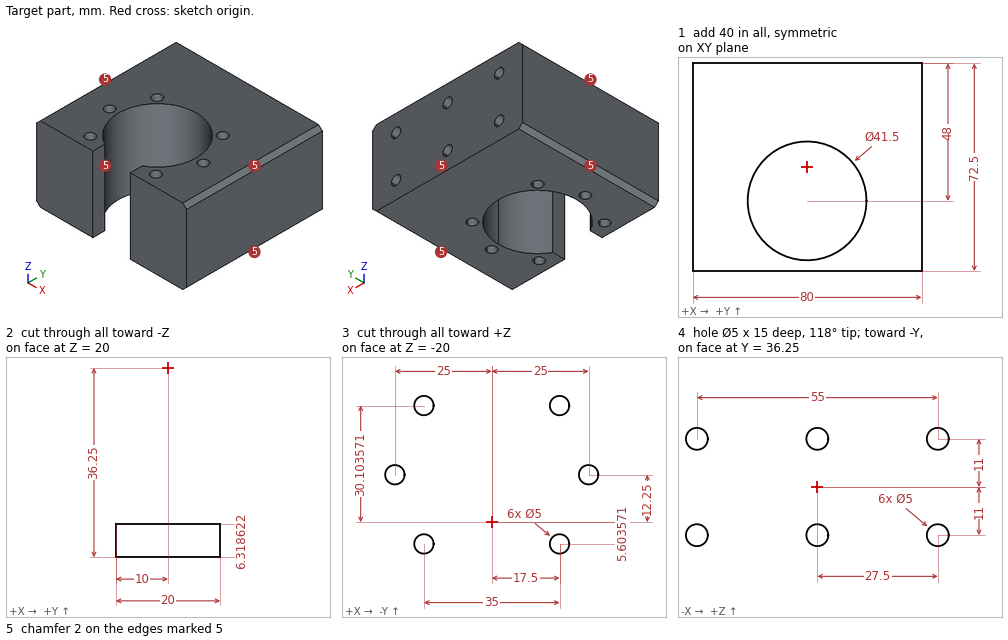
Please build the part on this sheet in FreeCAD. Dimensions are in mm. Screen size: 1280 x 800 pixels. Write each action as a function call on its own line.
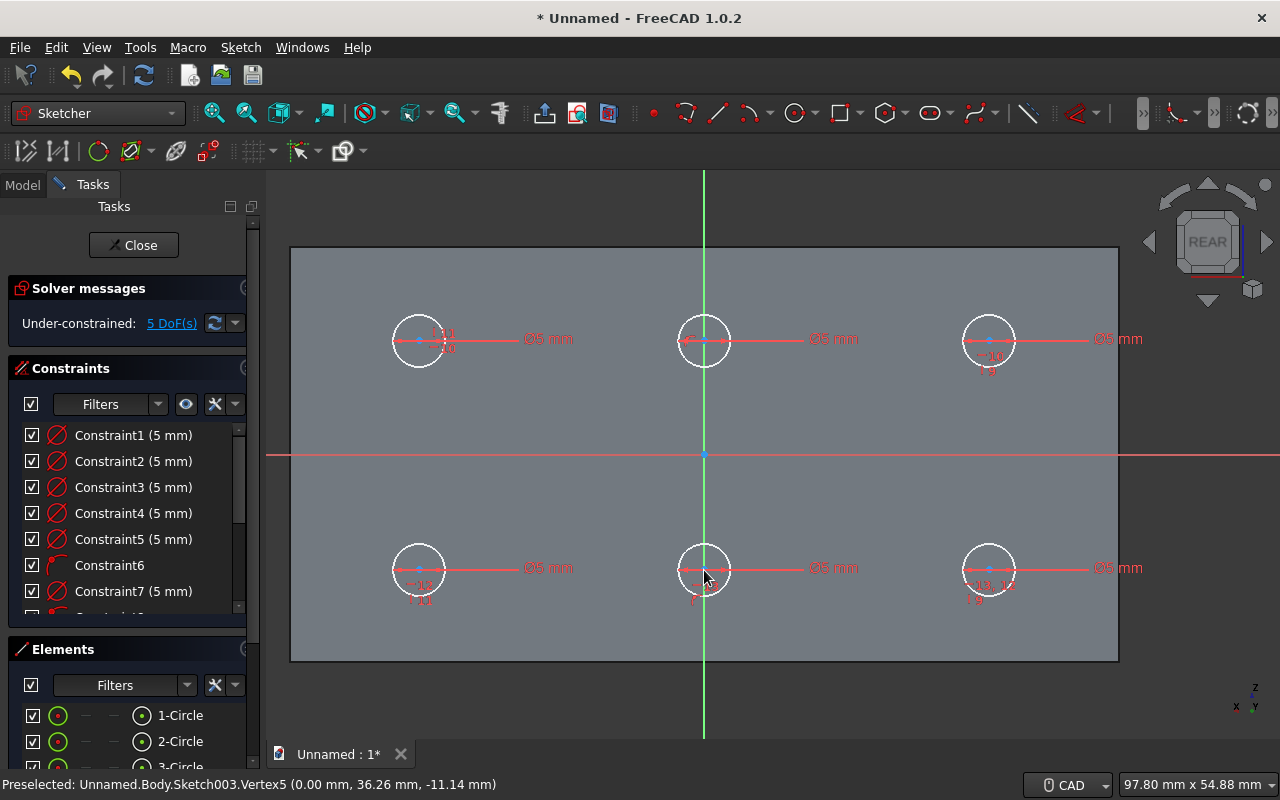
click(989, 341)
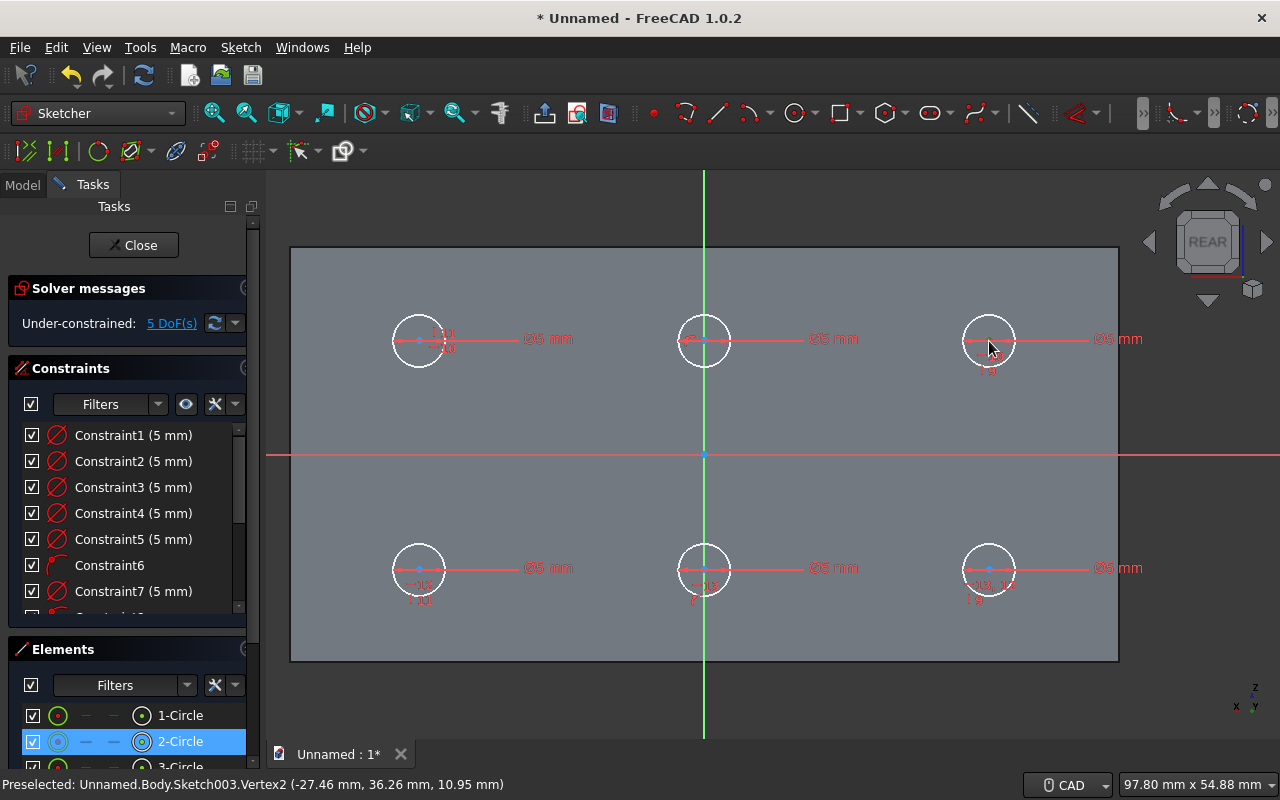
click(704, 341)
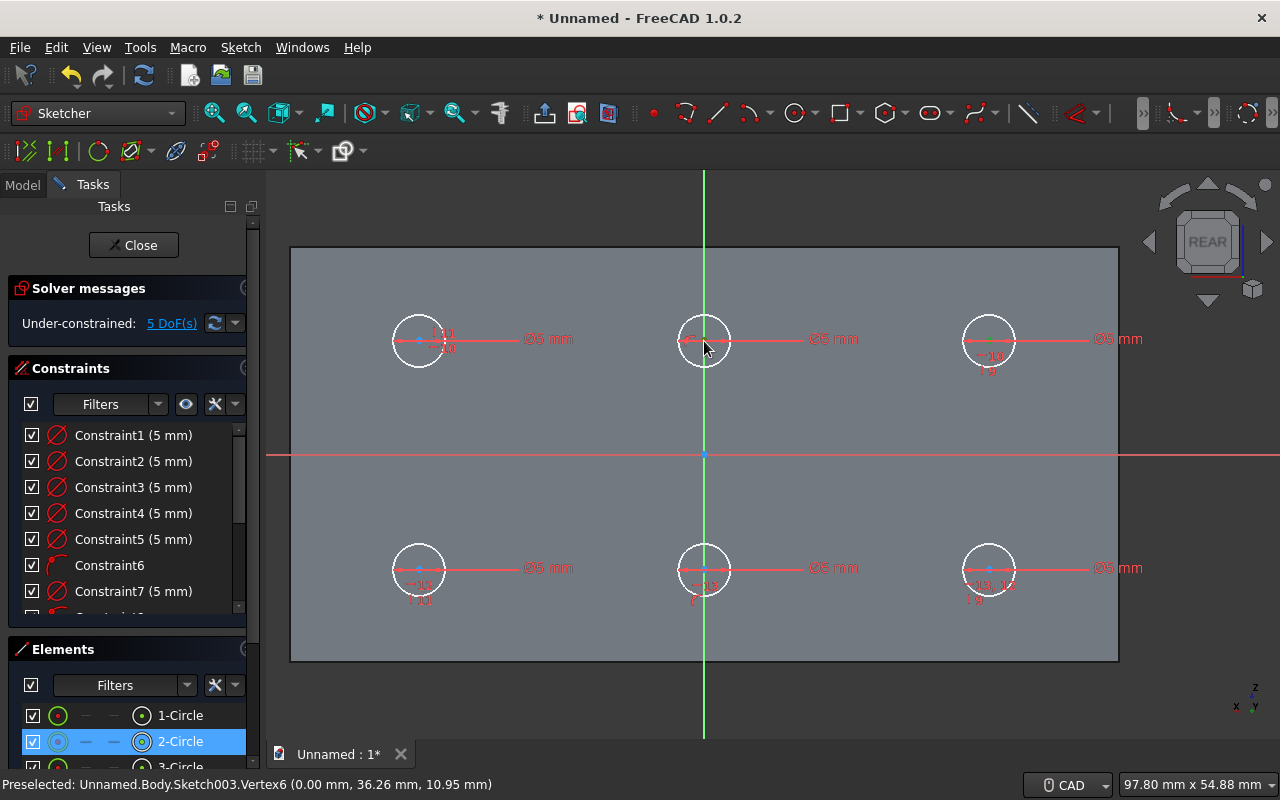
key(h)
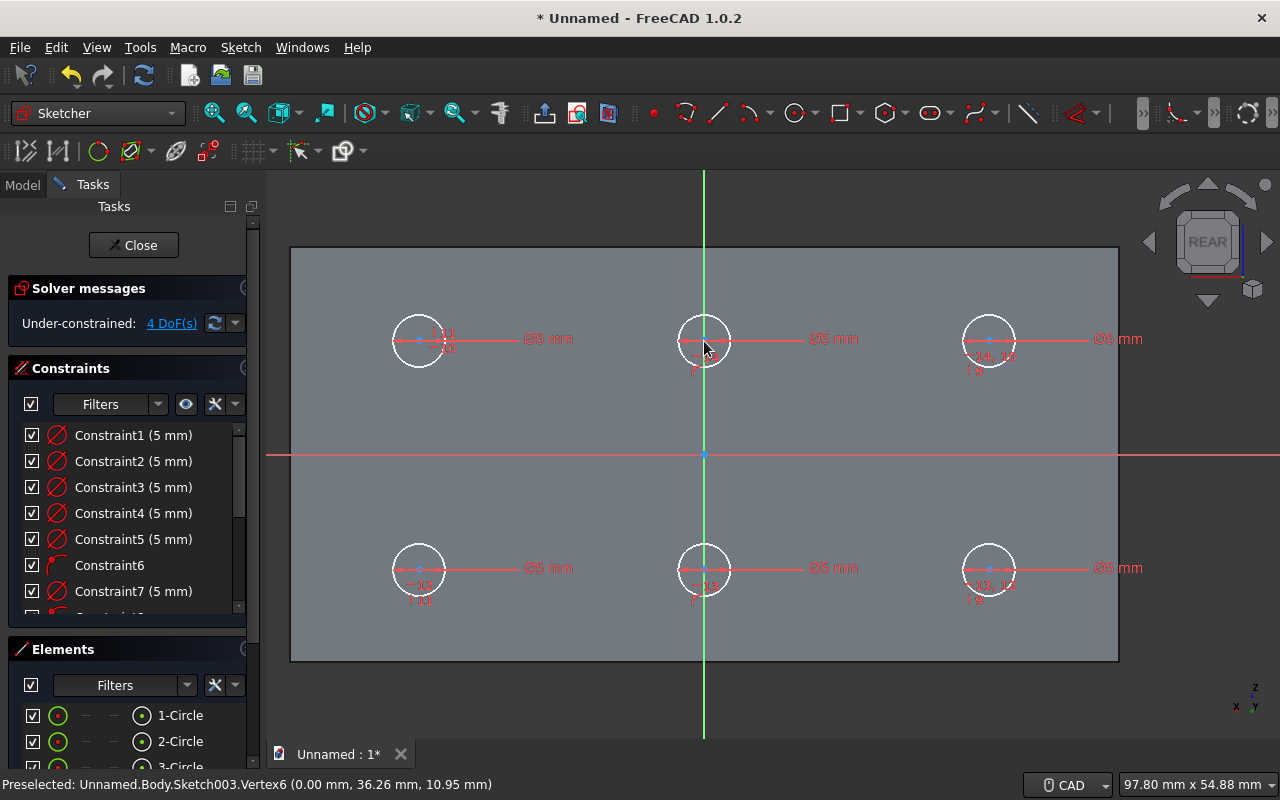
click(1076, 114)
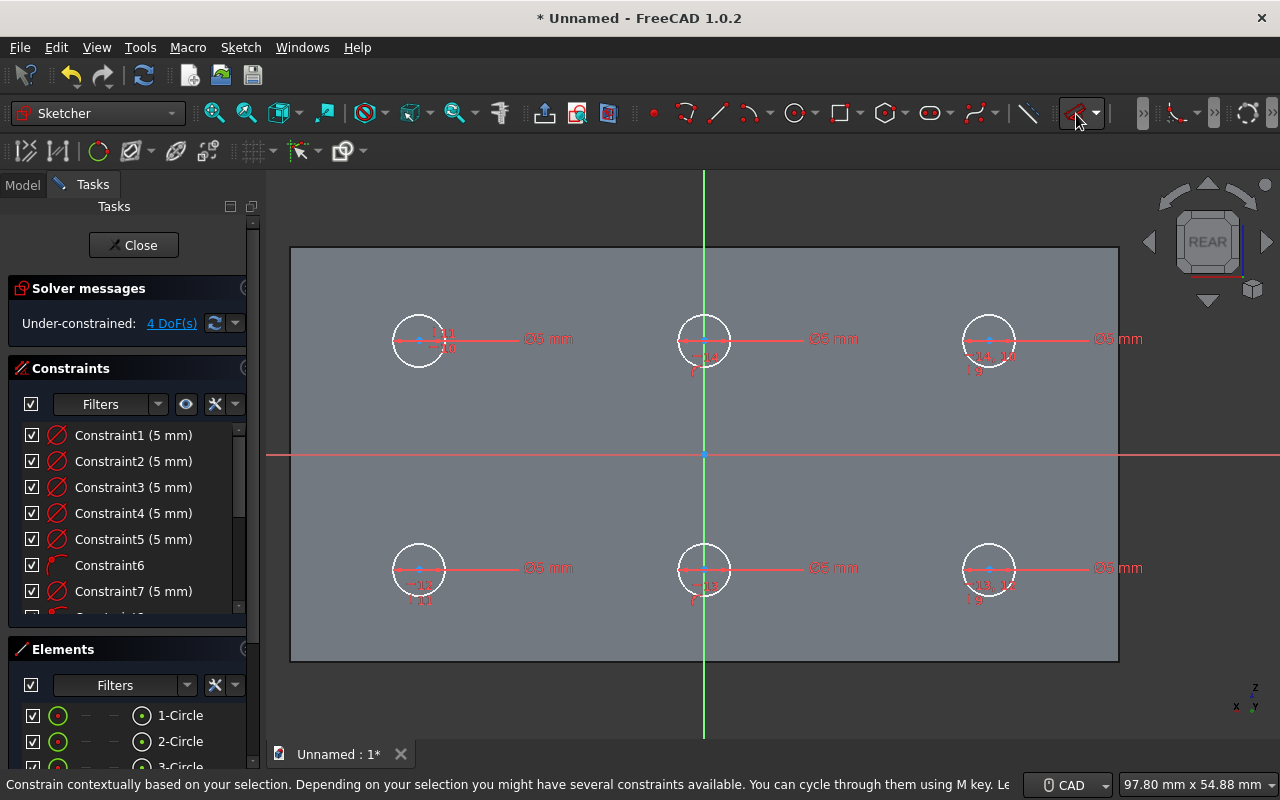
click(989, 570)
click(1023, 512)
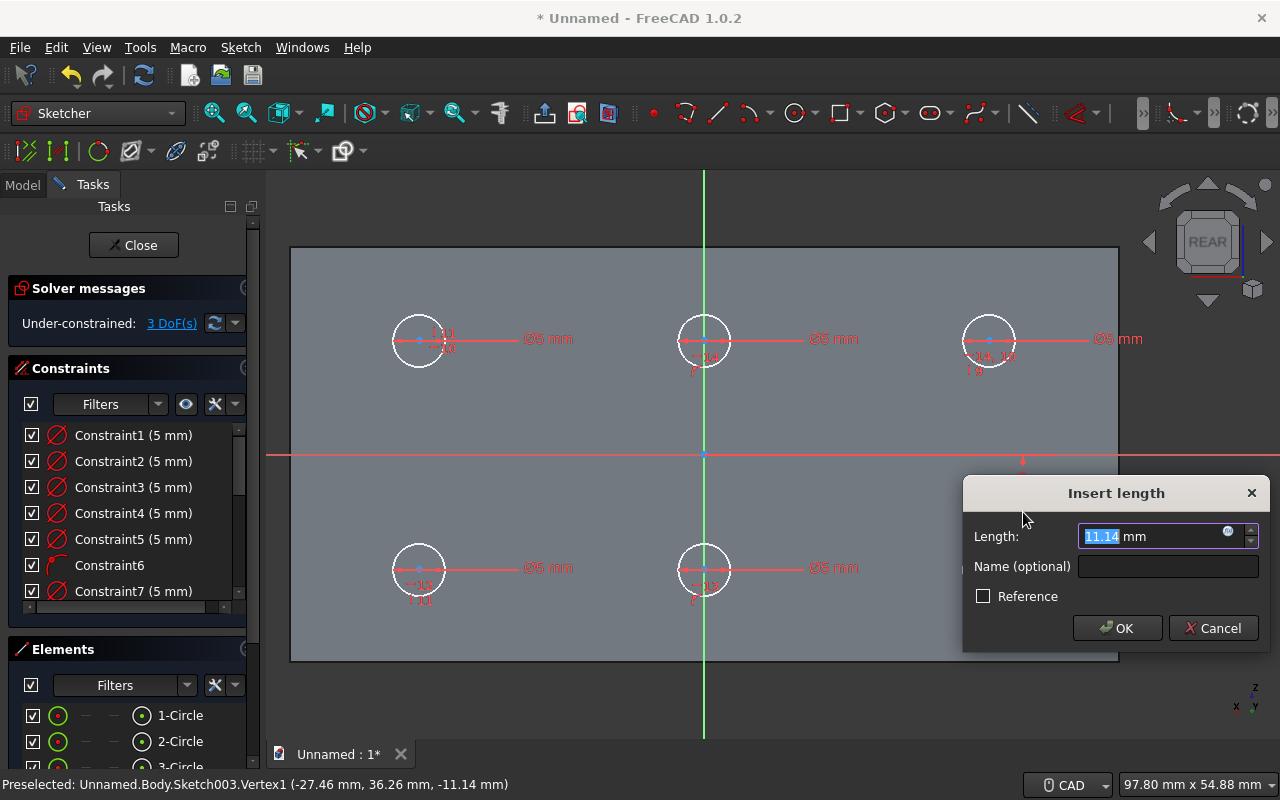
text(11)
key(Return)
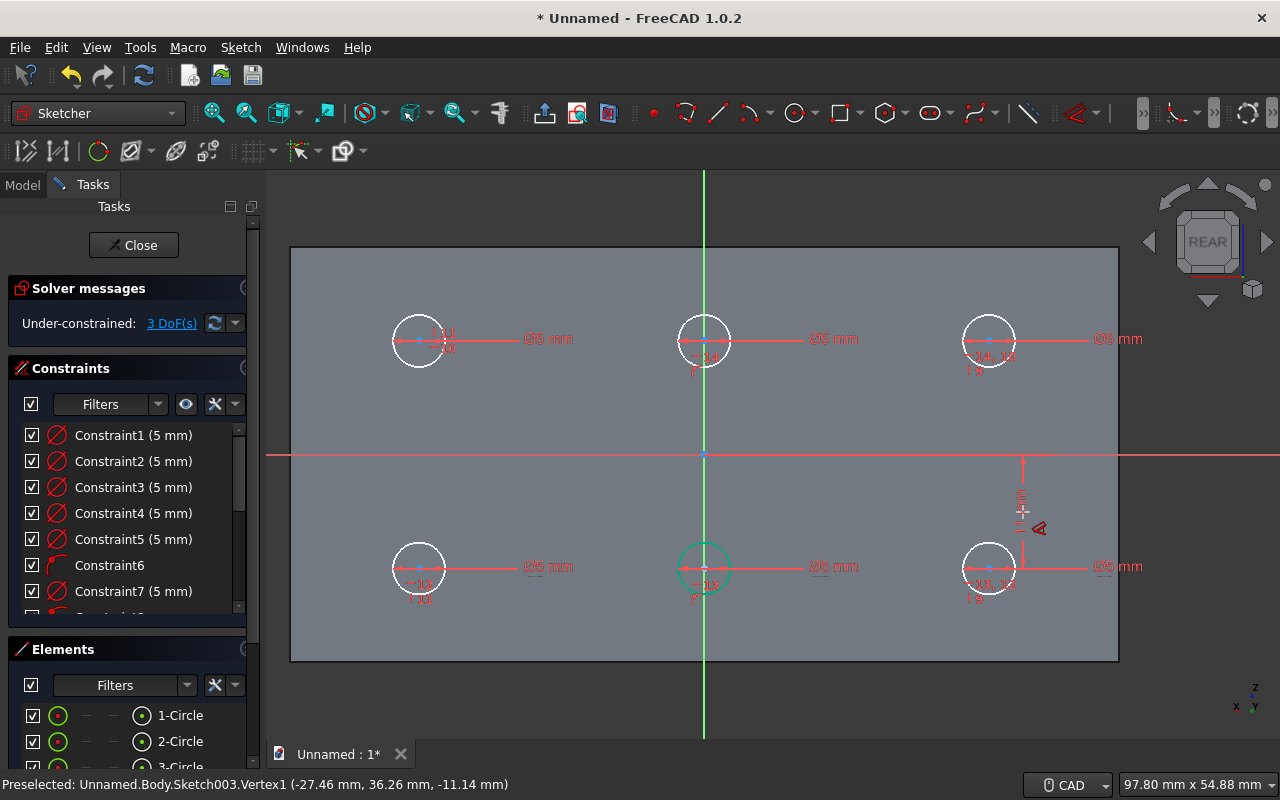
click(989, 341)
click(1023, 398)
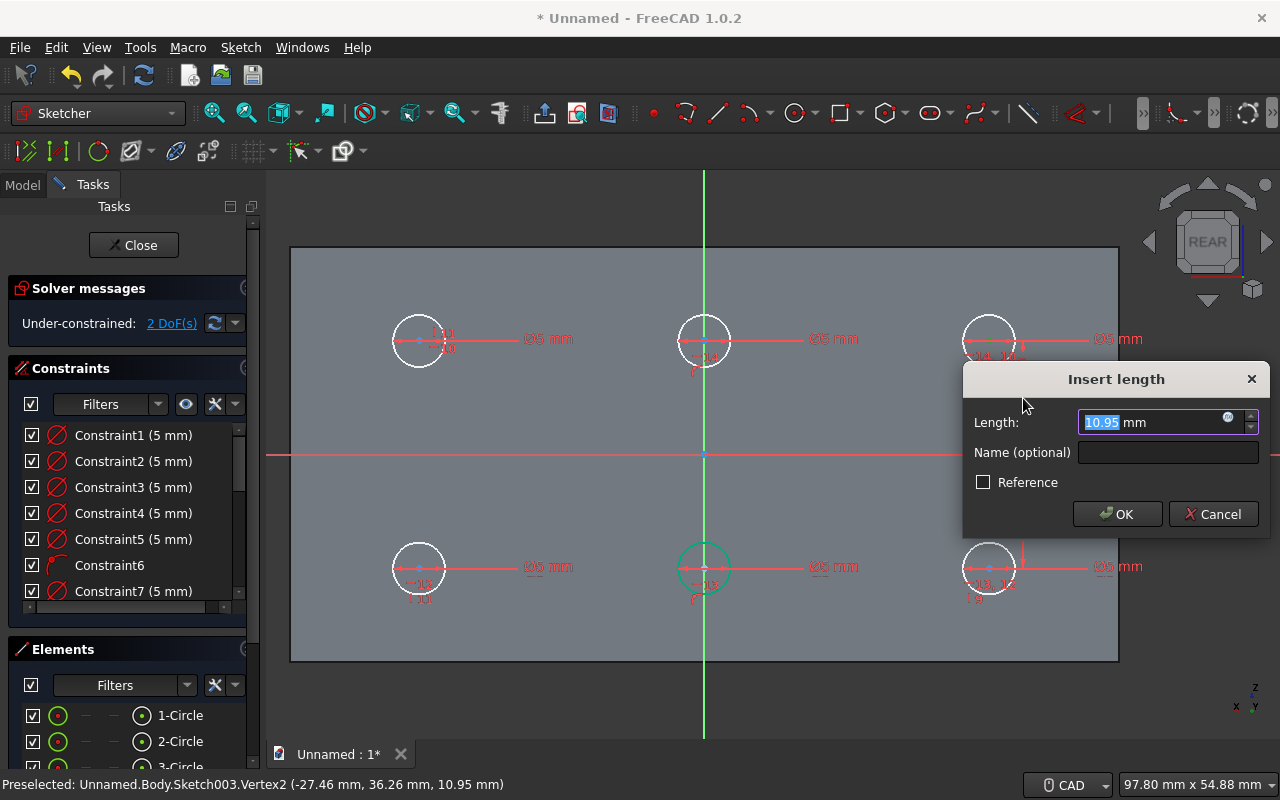
text(11)
key(Return)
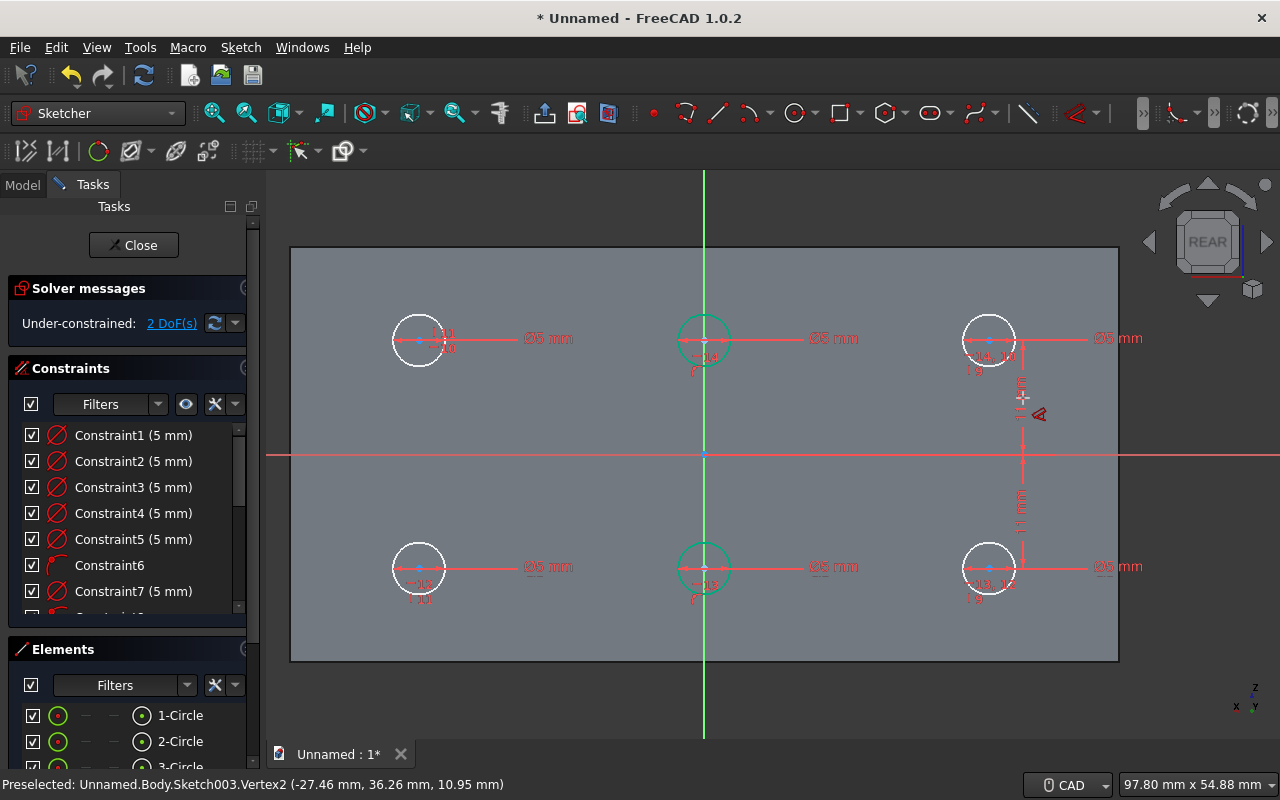
click(989, 340)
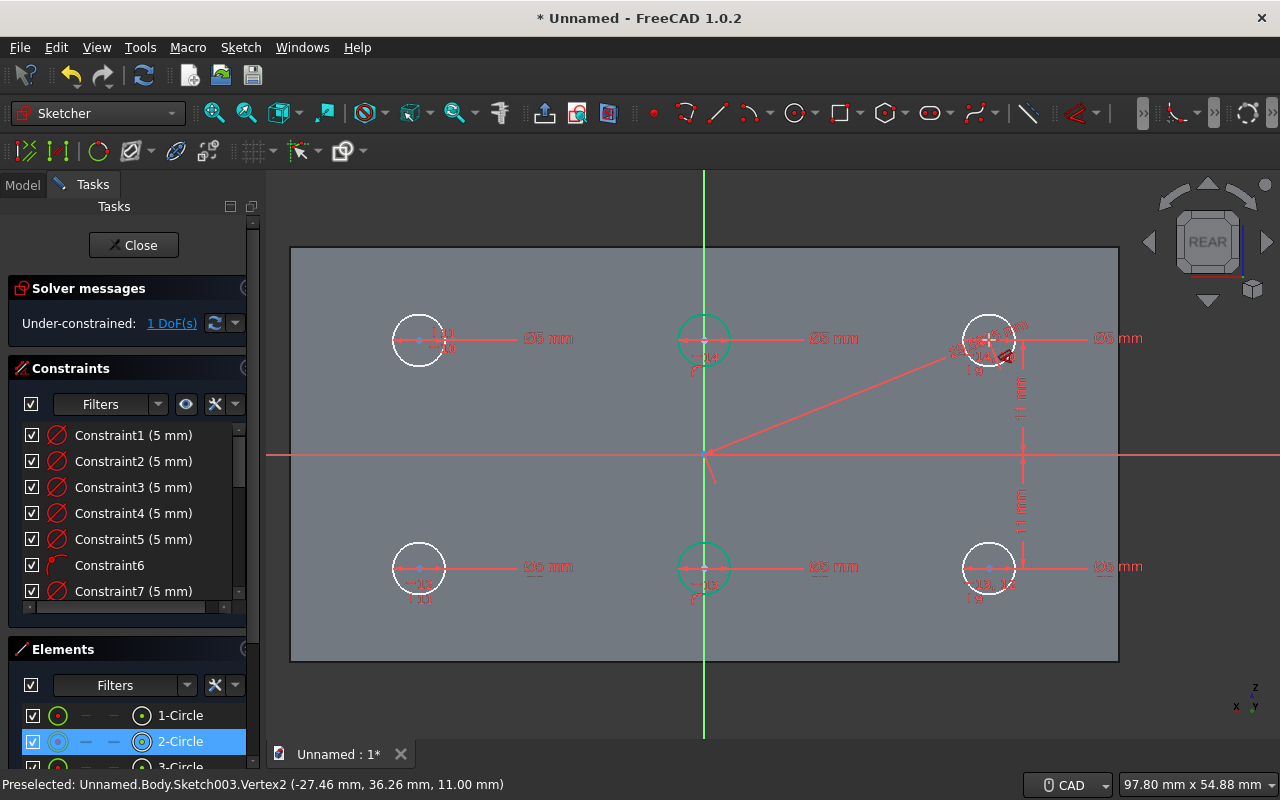
click(419, 340)
click(573, 306)